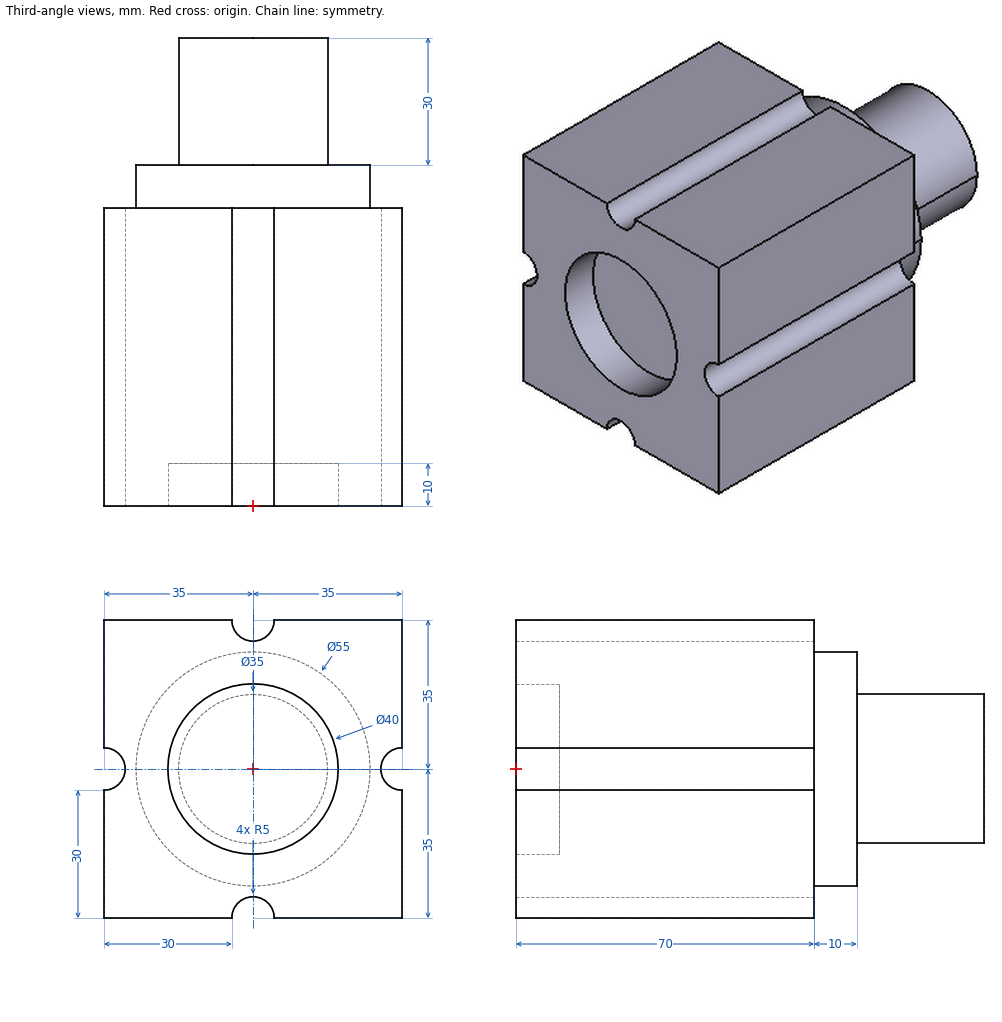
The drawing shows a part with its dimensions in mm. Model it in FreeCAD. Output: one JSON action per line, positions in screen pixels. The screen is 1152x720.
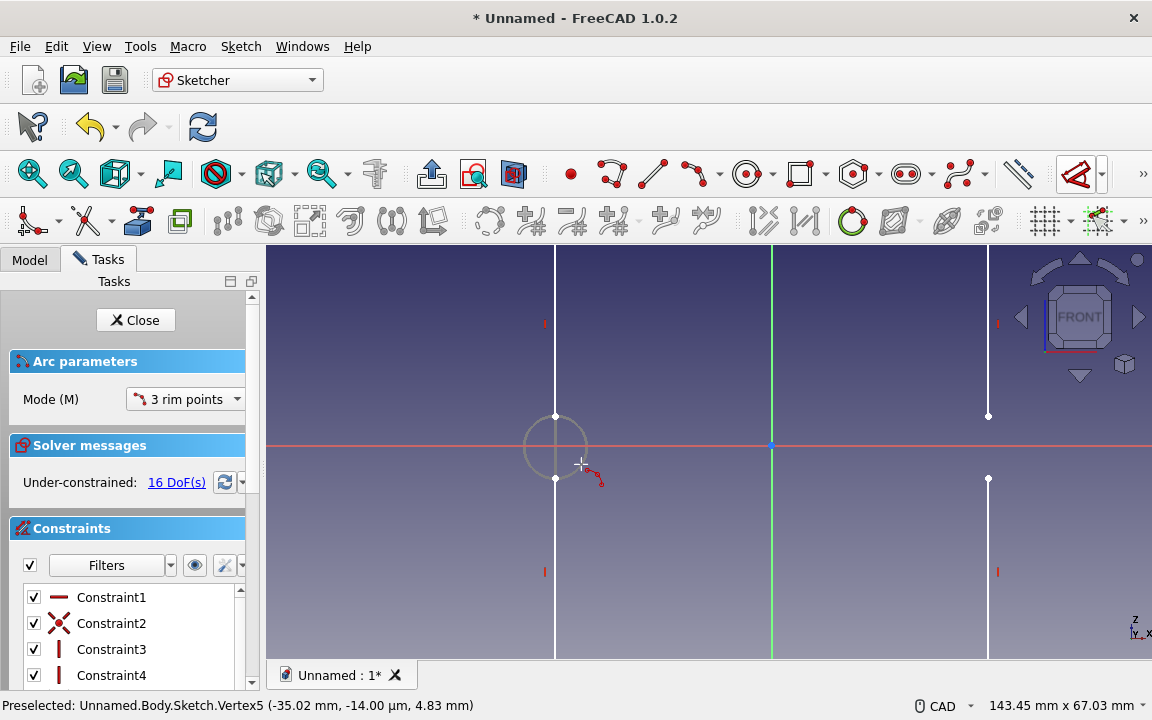
{"action": "left_click", "coordinate": [581, 464]}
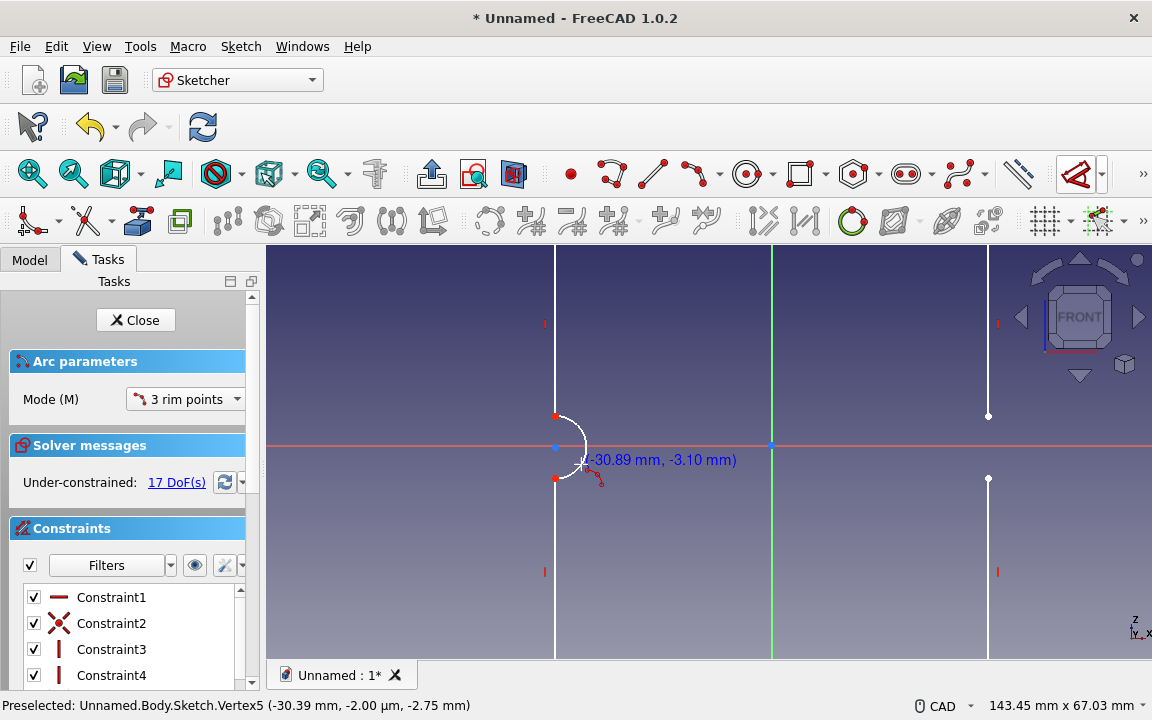
{"action": "scroll", "coordinate": [481, 459], "scroll_direction": "down", "scroll_amount": 3}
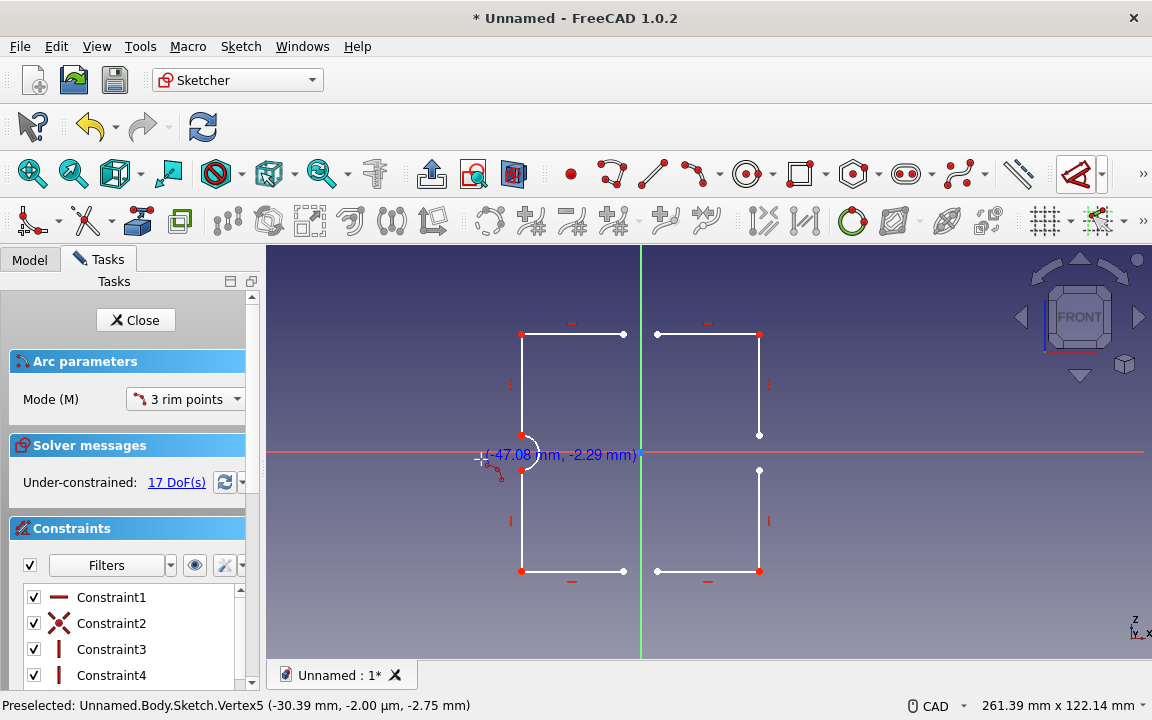
{"action": "left_click", "coordinate": [623, 334]}
{"action": "left_click", "coordinate": [658, 334]}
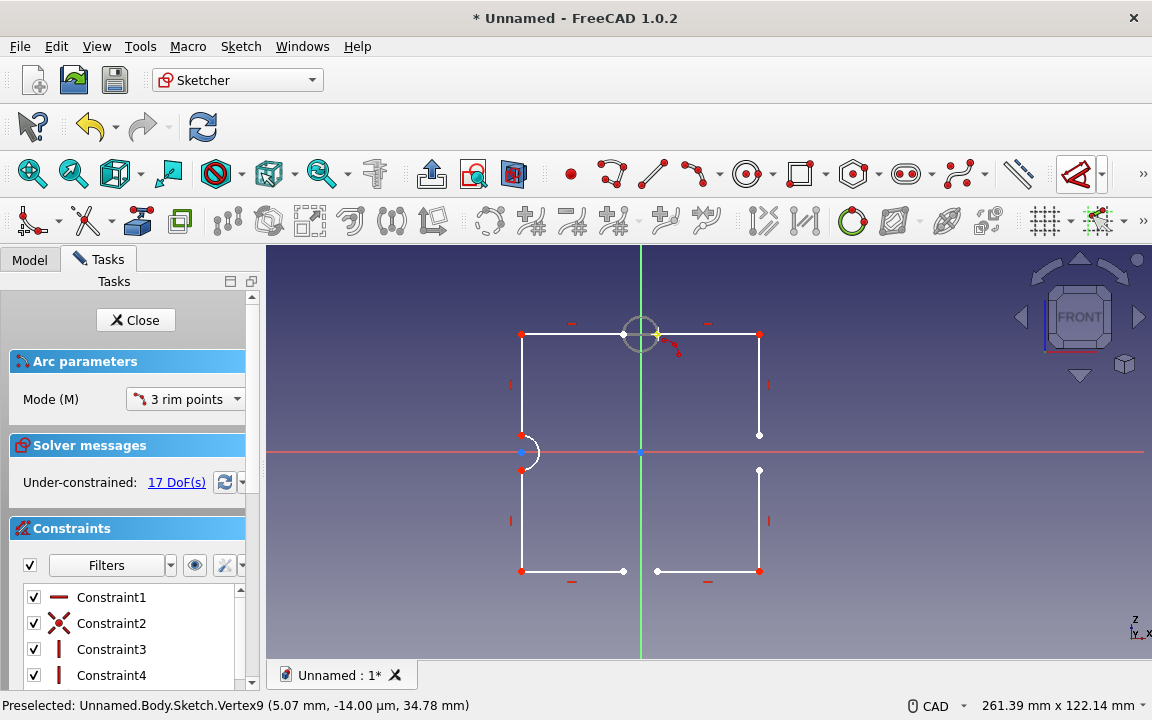
{"action": "scroll", "coordinate": [631, 347], "scroll_direction": "up", "scroll_amount": 3}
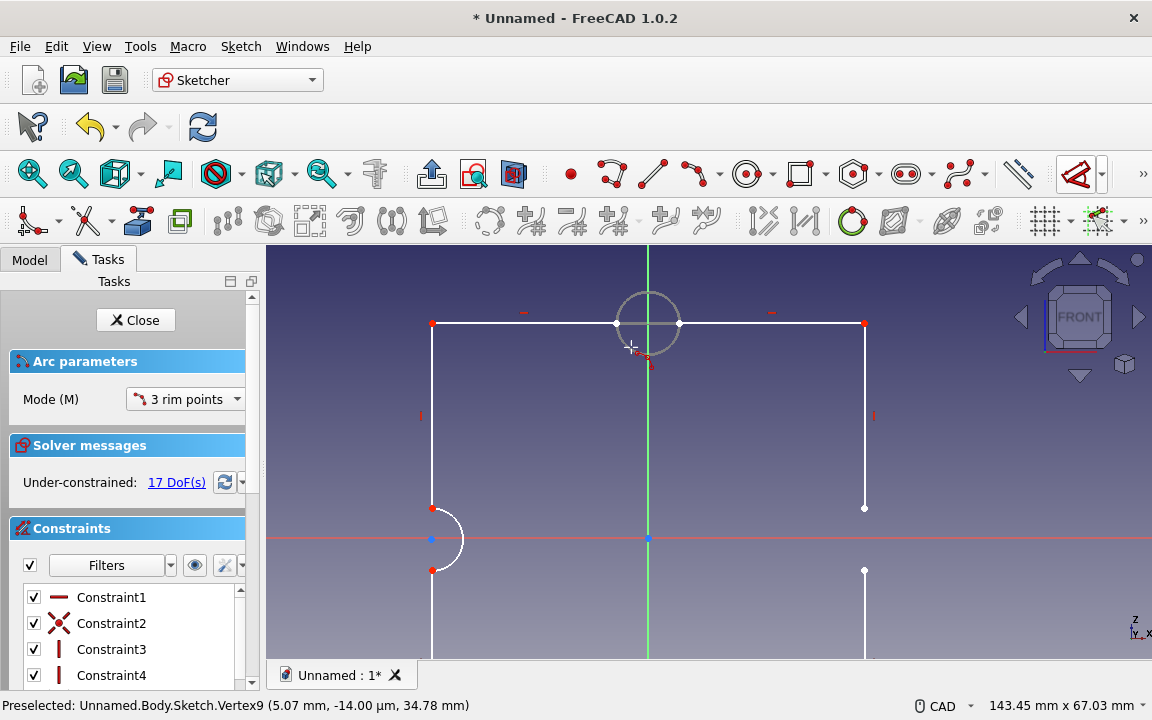
{"action": "left_click", "coordinate": [630, 347]}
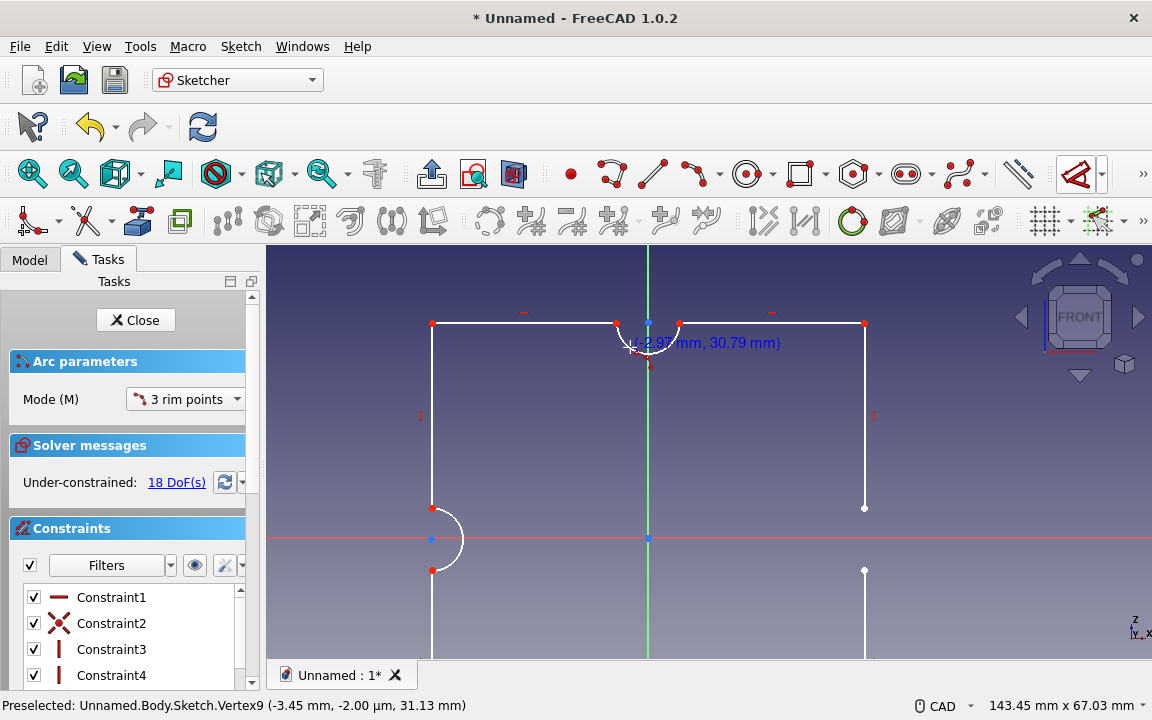
{"action": "left_click", "coordinate": [865, 508]}
{"action": "left_click", "coordinate": [865, 571]}
{"action": "left_click", "coordinate": [840, 520]}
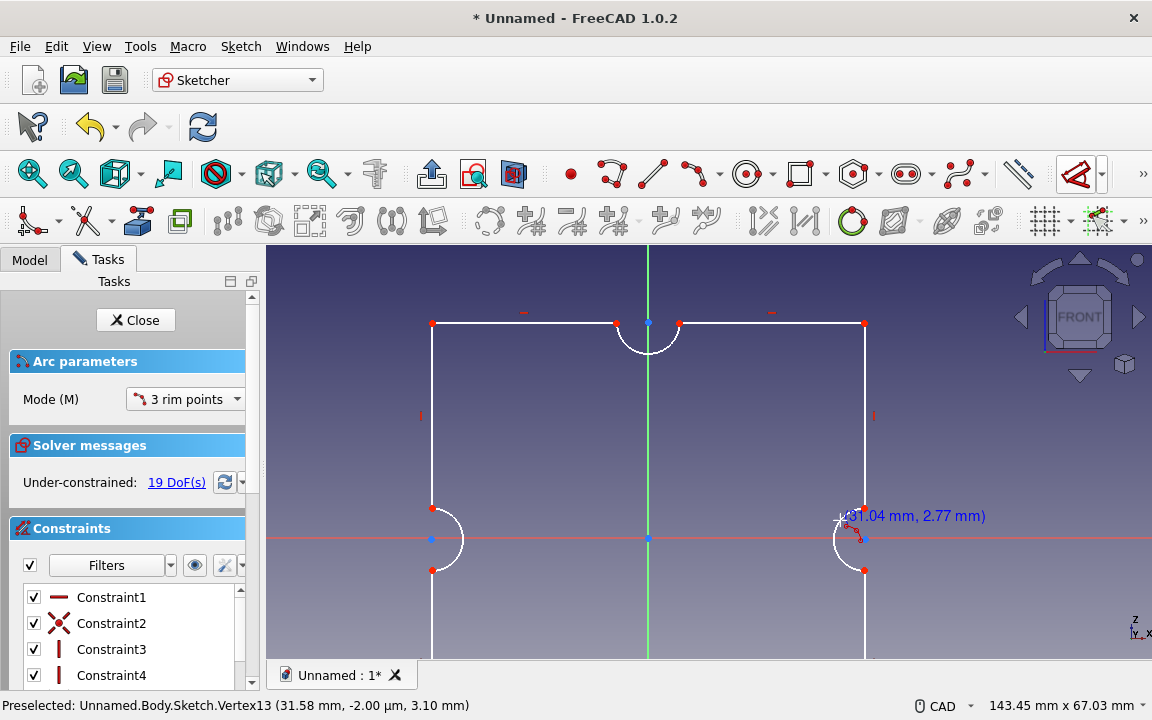
{"action": "scroll", "coordinate": [631, 347], "scroll_direction": "down", "scroll_amount": 3}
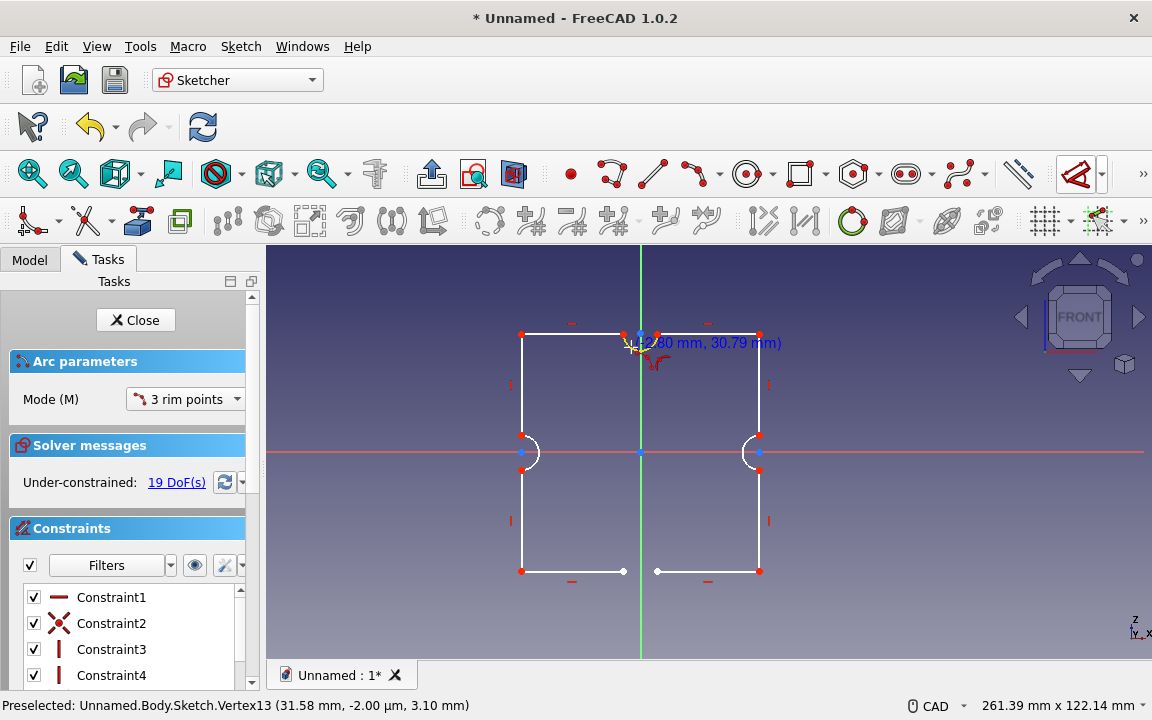
{"action": "left_click", "coordinate": [658, 572]}
{"action": "left_click", "coordinate": [623, 572]}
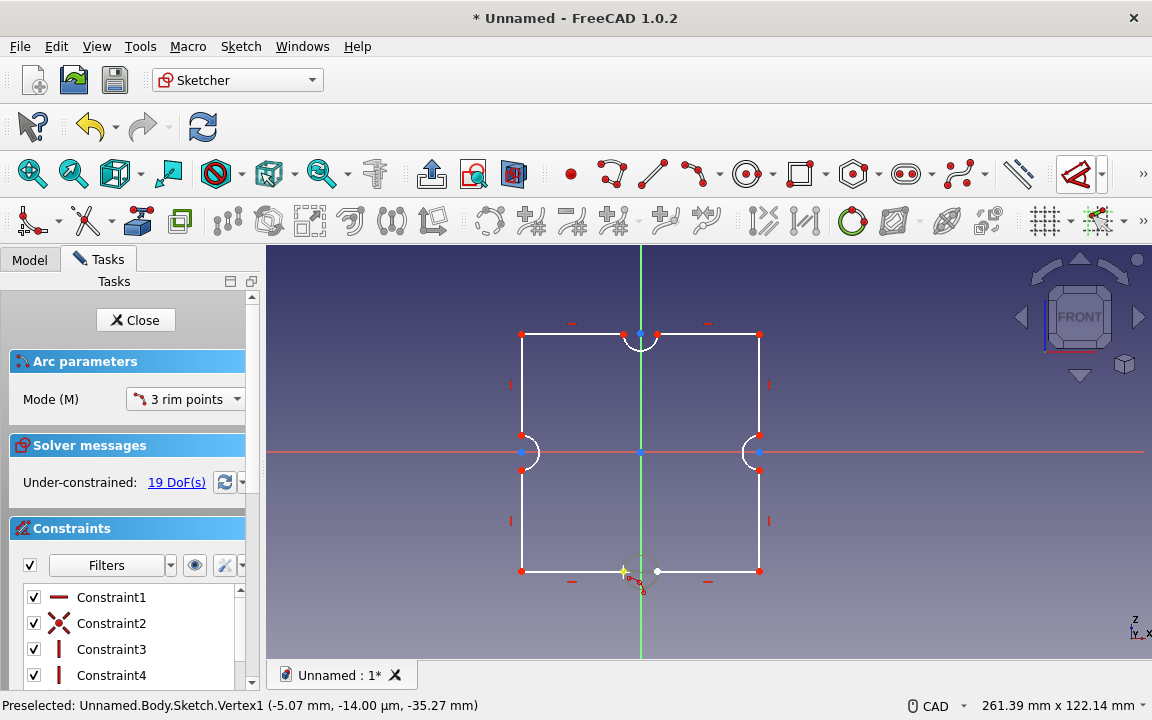
{"action": "scroll", "coordinate": [651, 557], "scroll_direction": "up", "scroll_amount": 3}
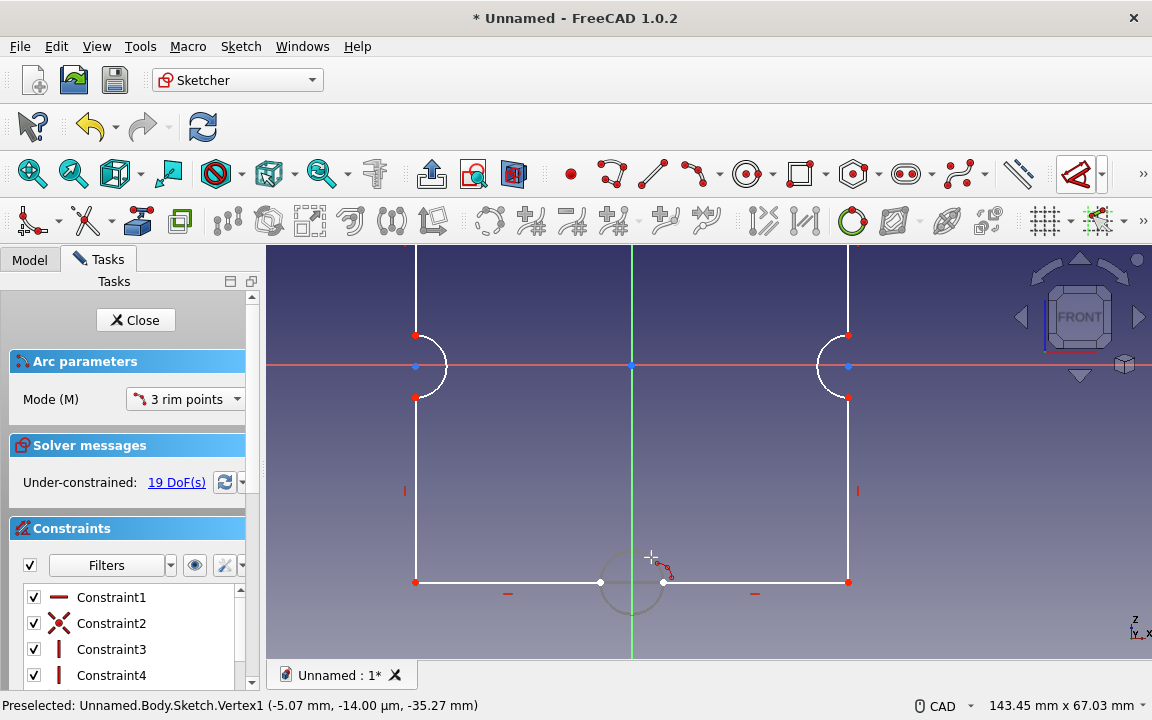
{"action": "left_click", "coordinate": [650, 556]}
{"action": "key", "text": "Escape"}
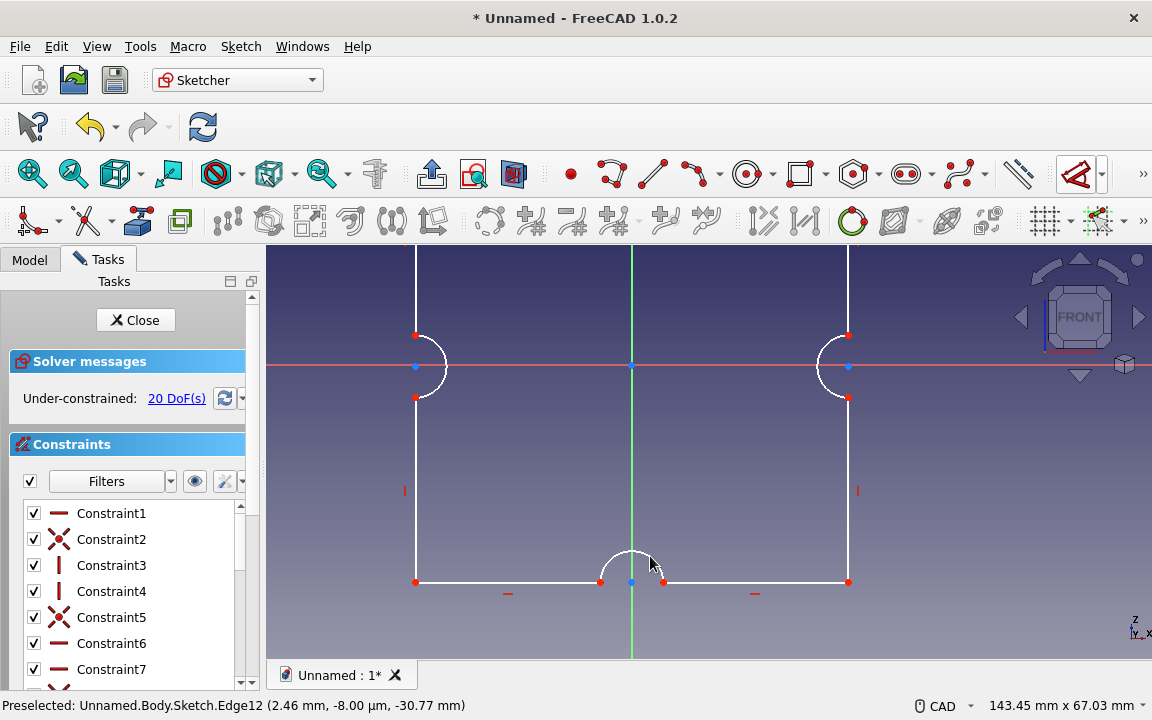
{"action": "left_click", "coordinate": [441, 385]}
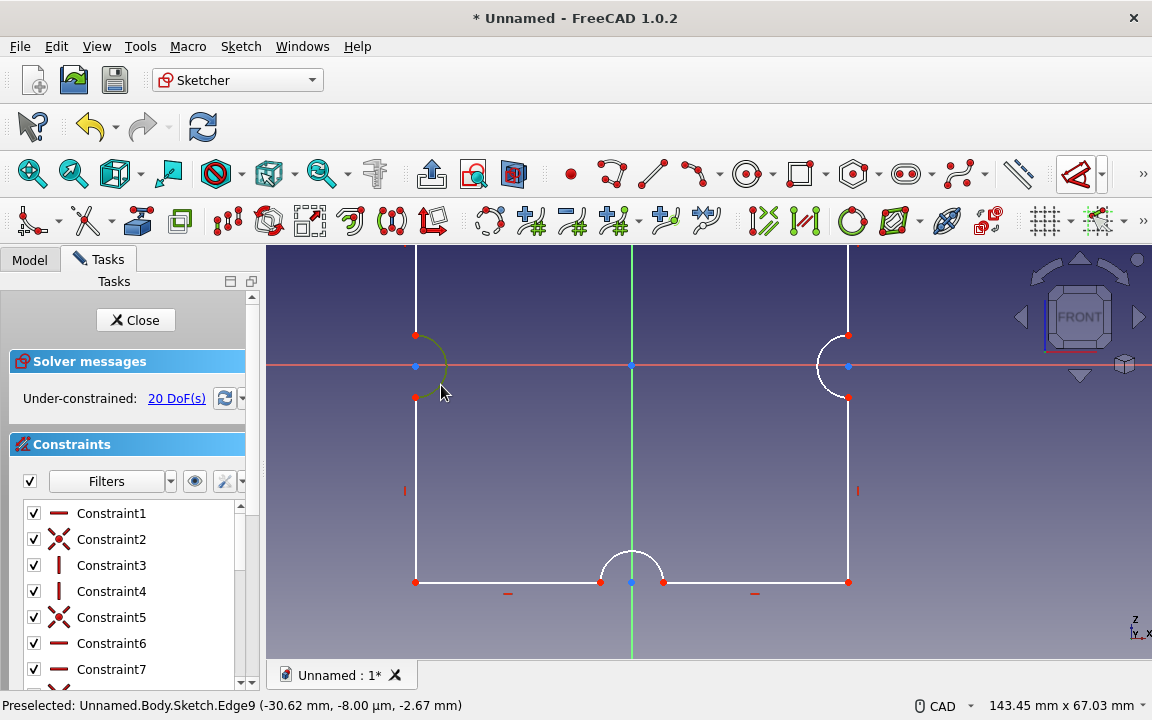
{"action": "scroll", "coordinate": [651, 558], "scroll_direction": "down", "scroll_amount": 3}